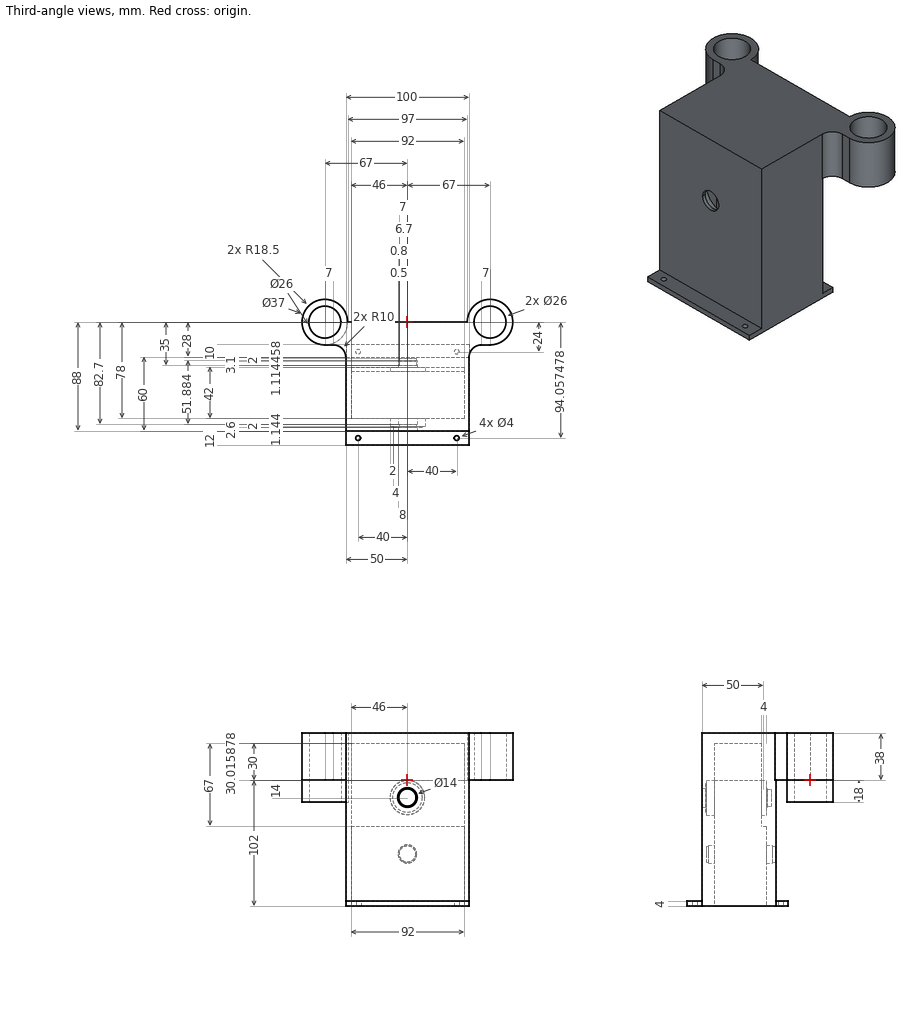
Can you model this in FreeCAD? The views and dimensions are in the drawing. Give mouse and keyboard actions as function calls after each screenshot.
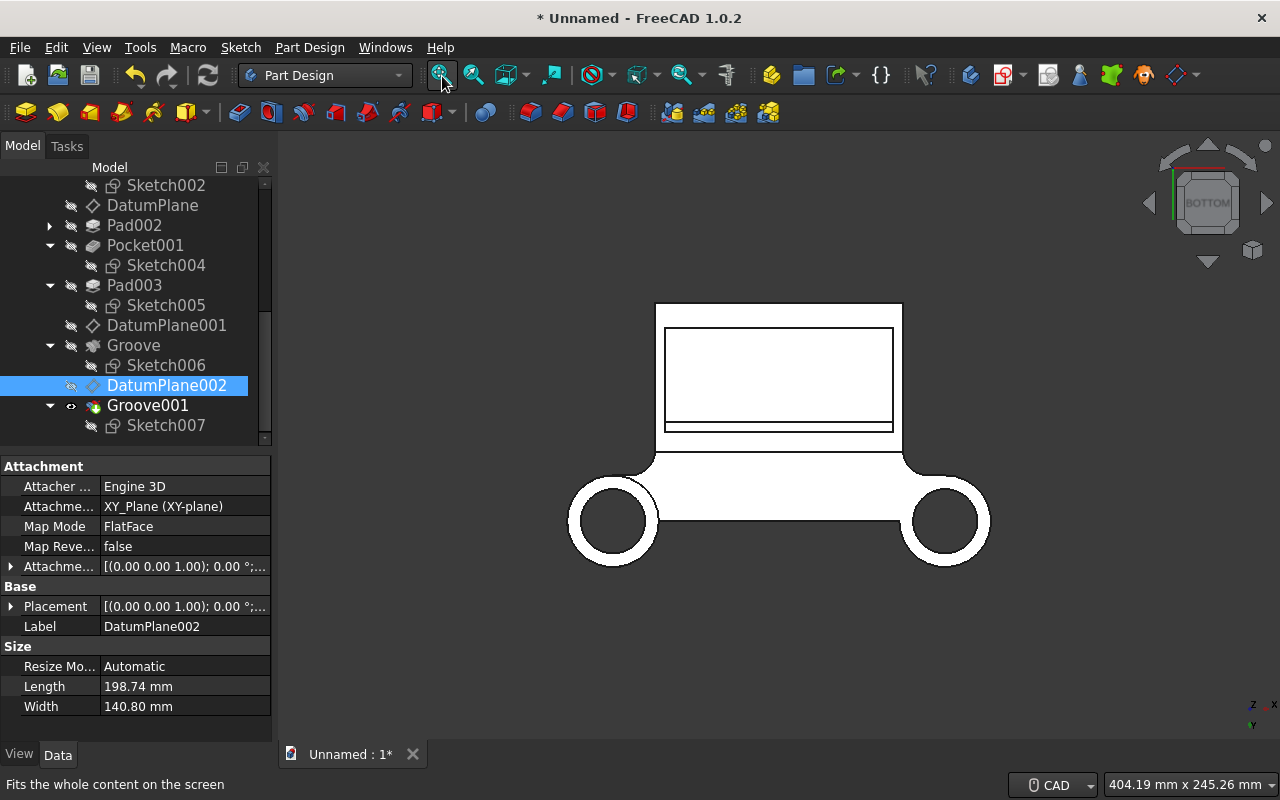
click(885, 313)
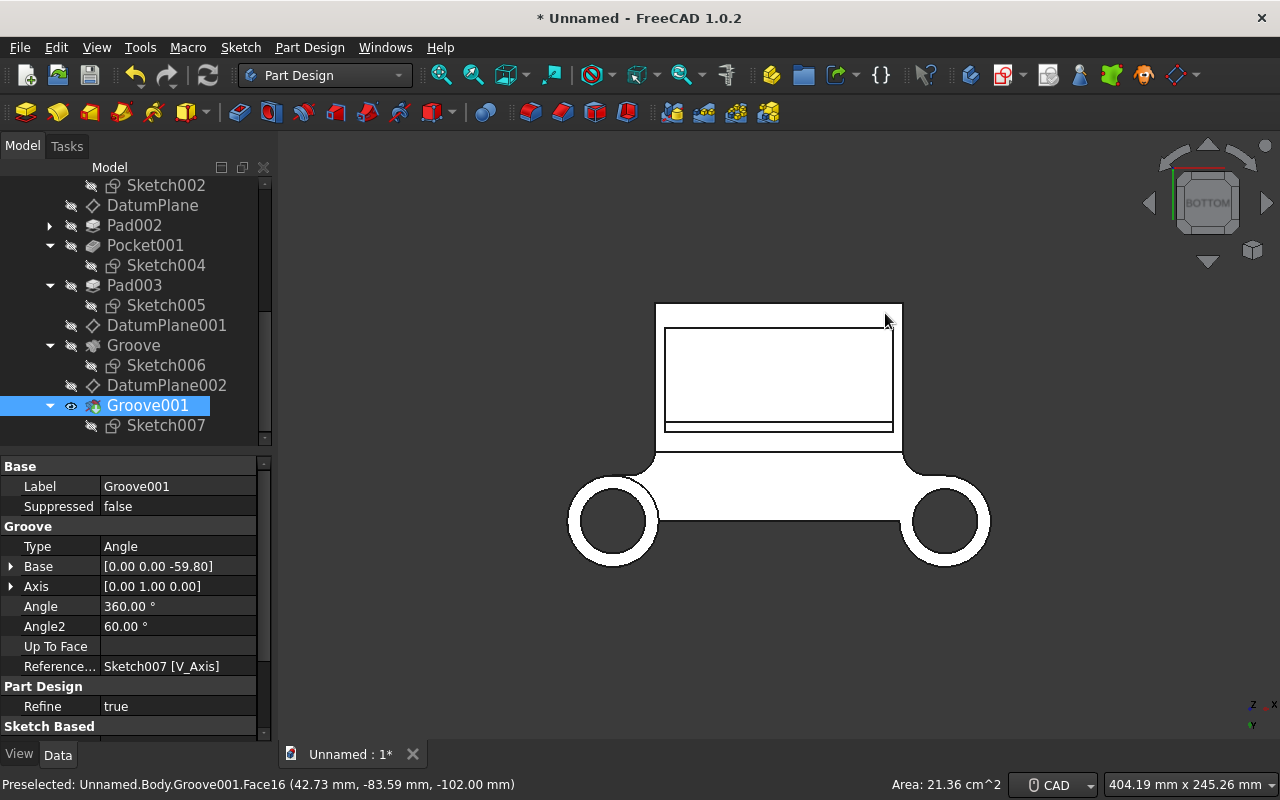
click(1004, 76)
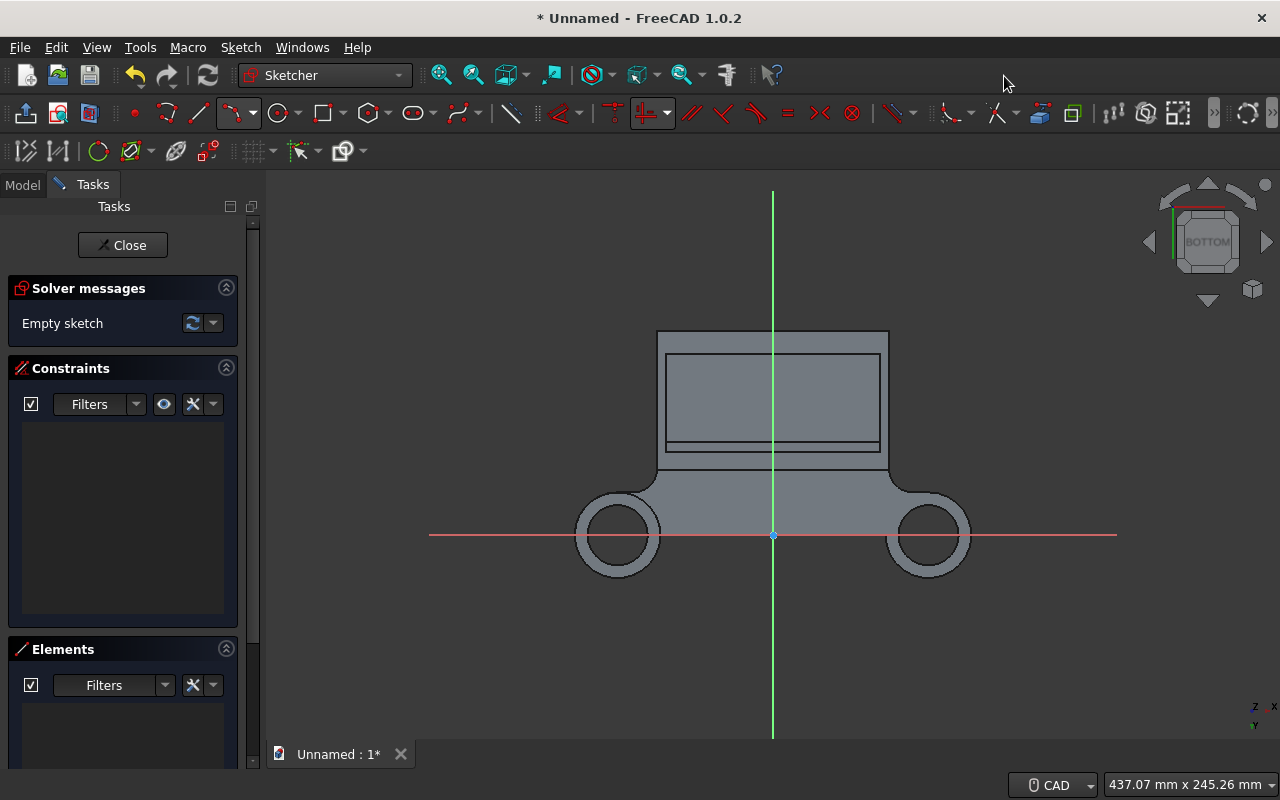
scroll(912, 347, up, 2)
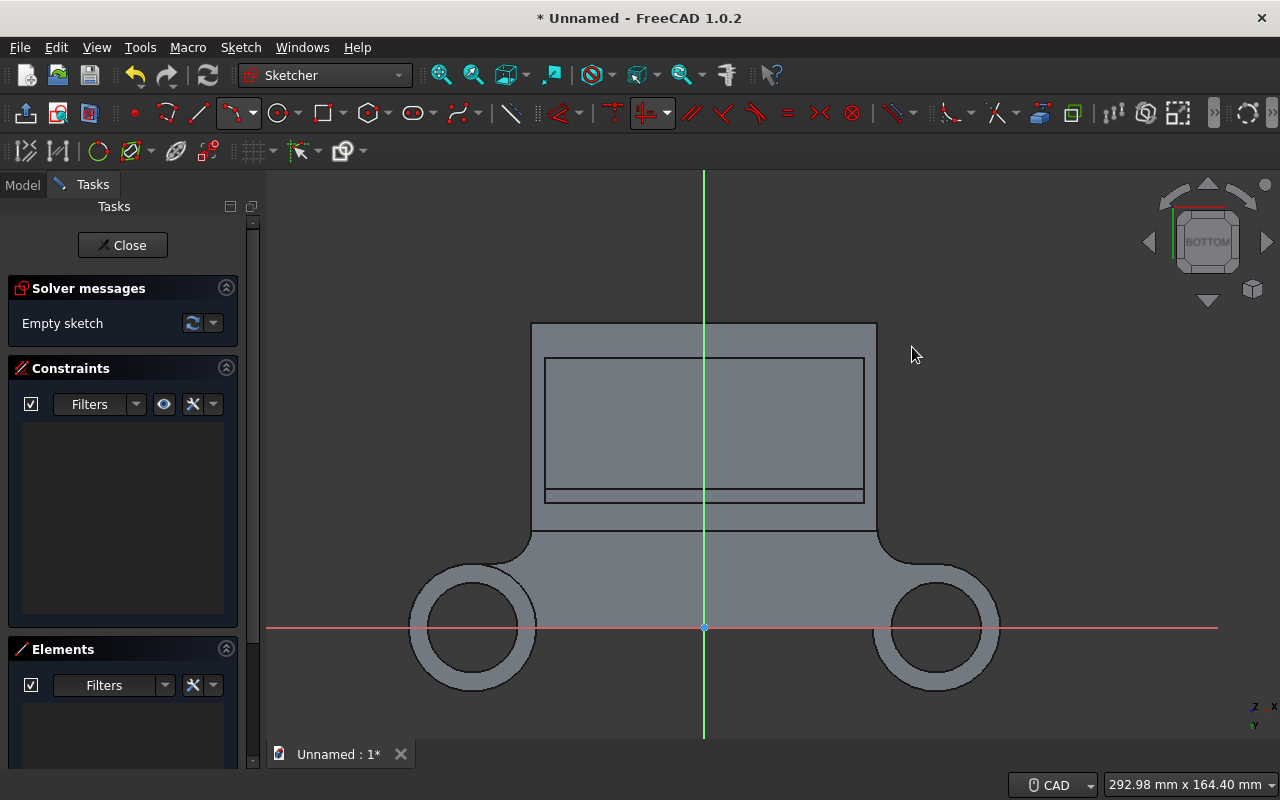
key(g)
key(r)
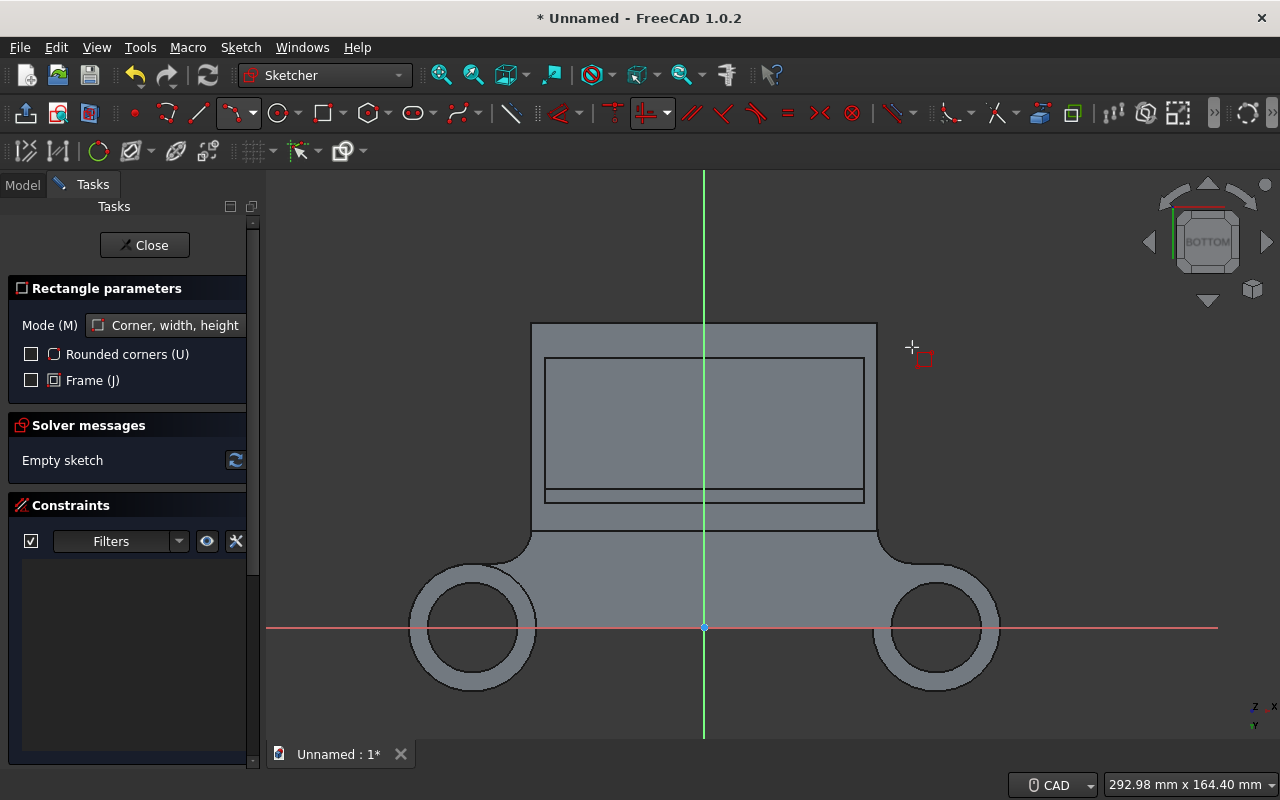
click(531, 531)
click(877, 565)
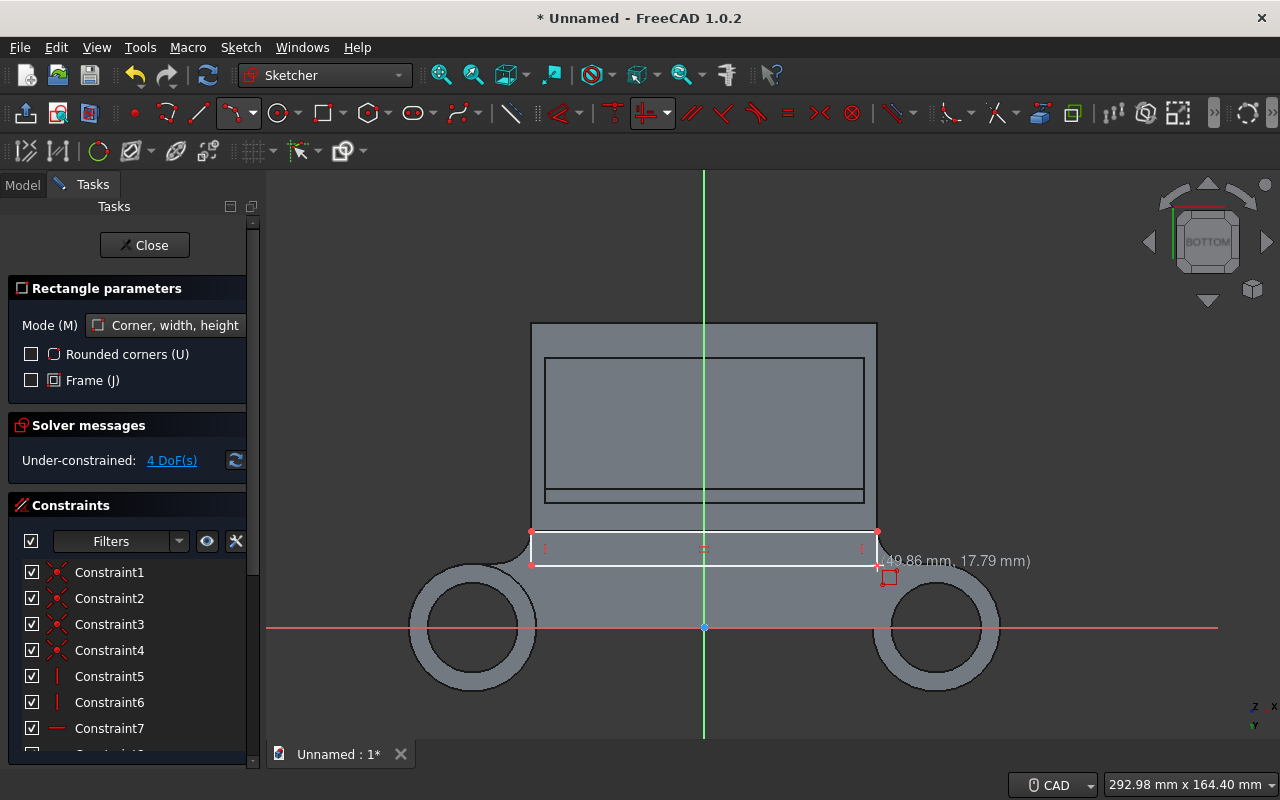
click(531, 281)
click(877, 323)
key(Escape)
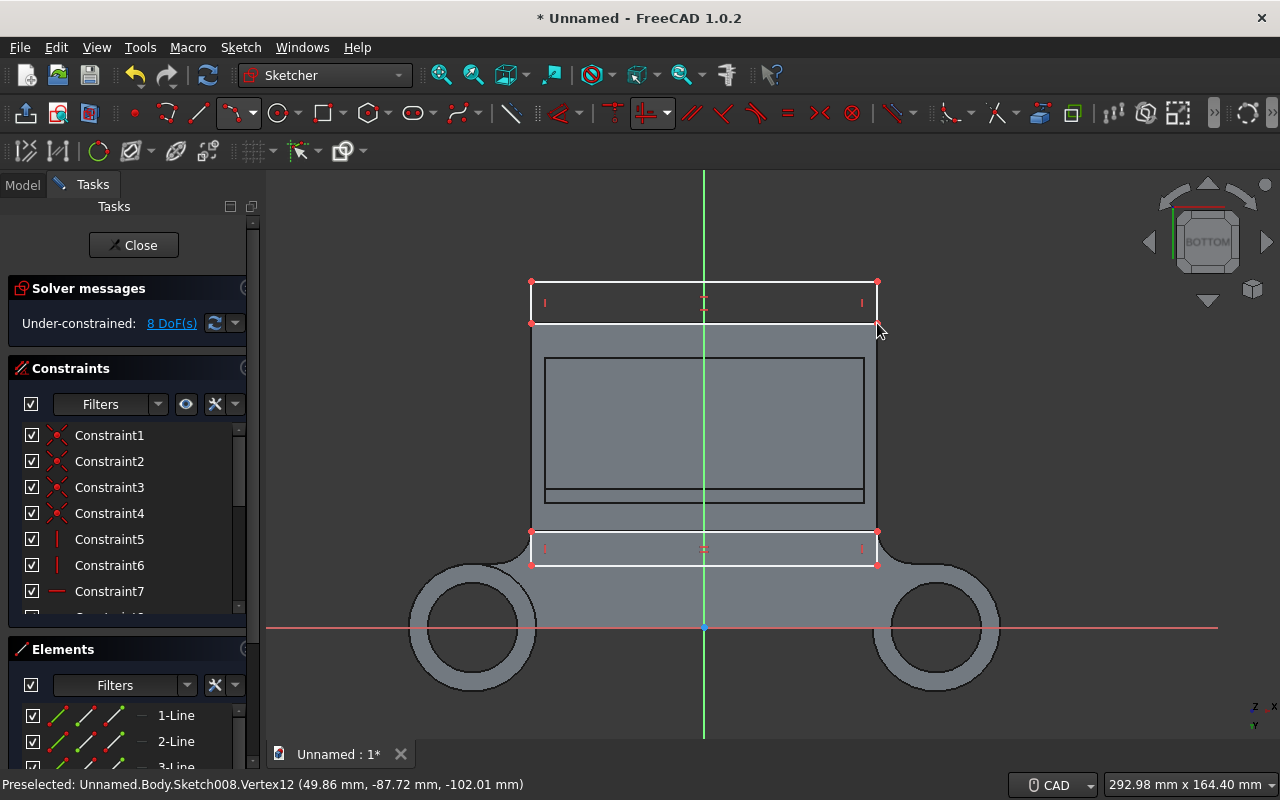
key(d)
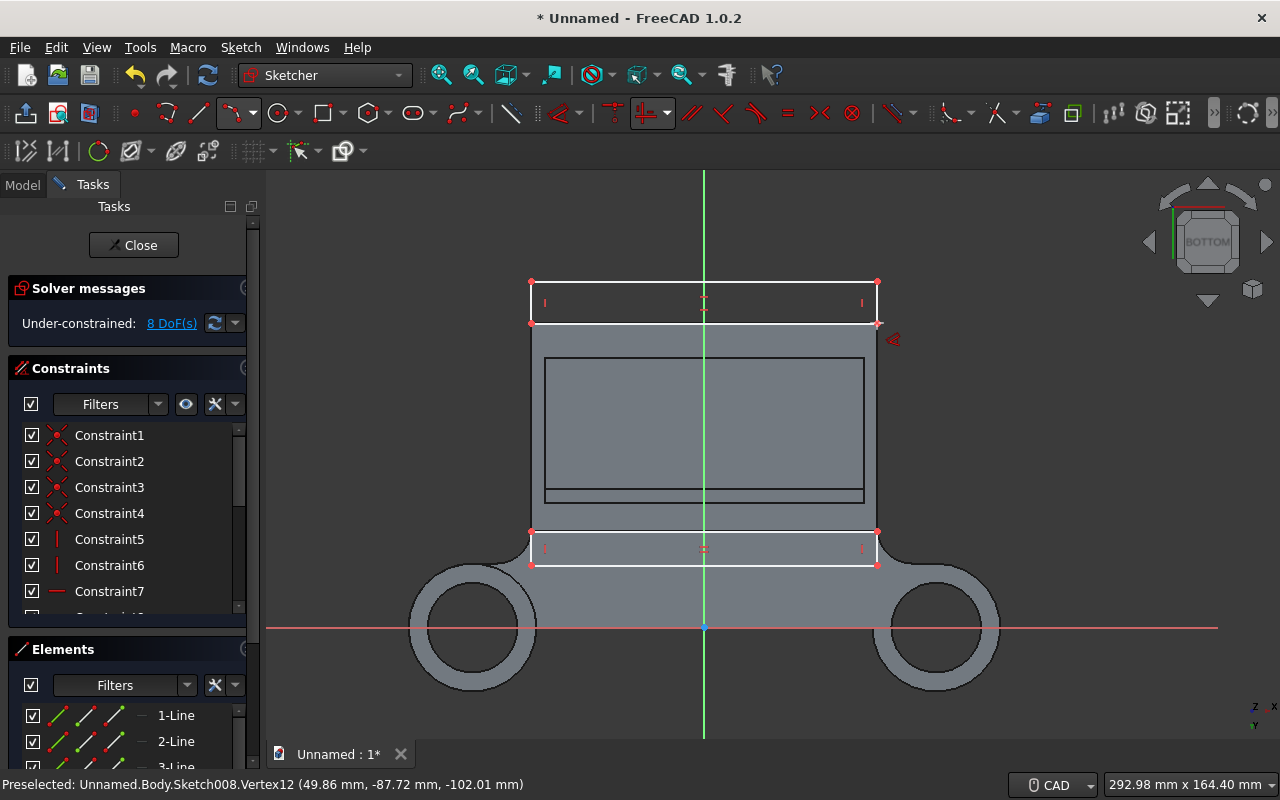
scroll(531, 542, up, 2)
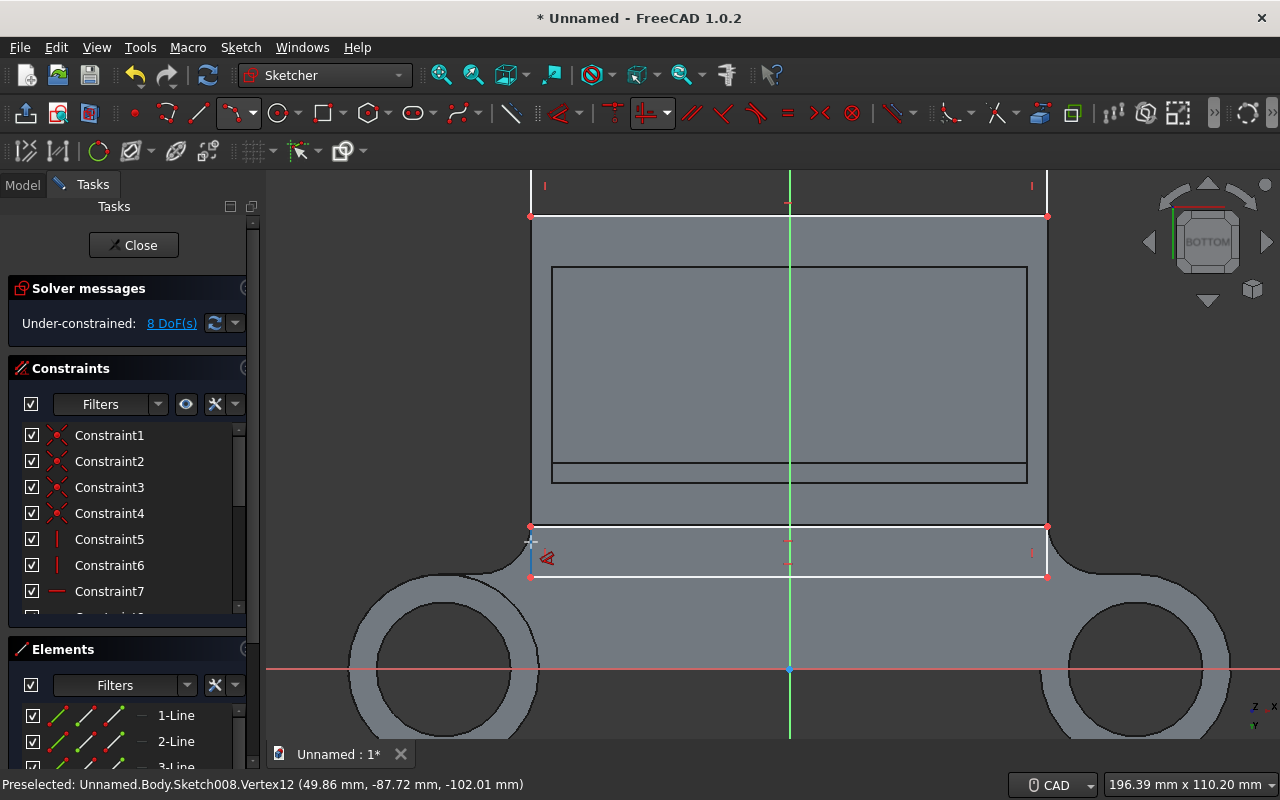
click(531, 542)
click(497, 552)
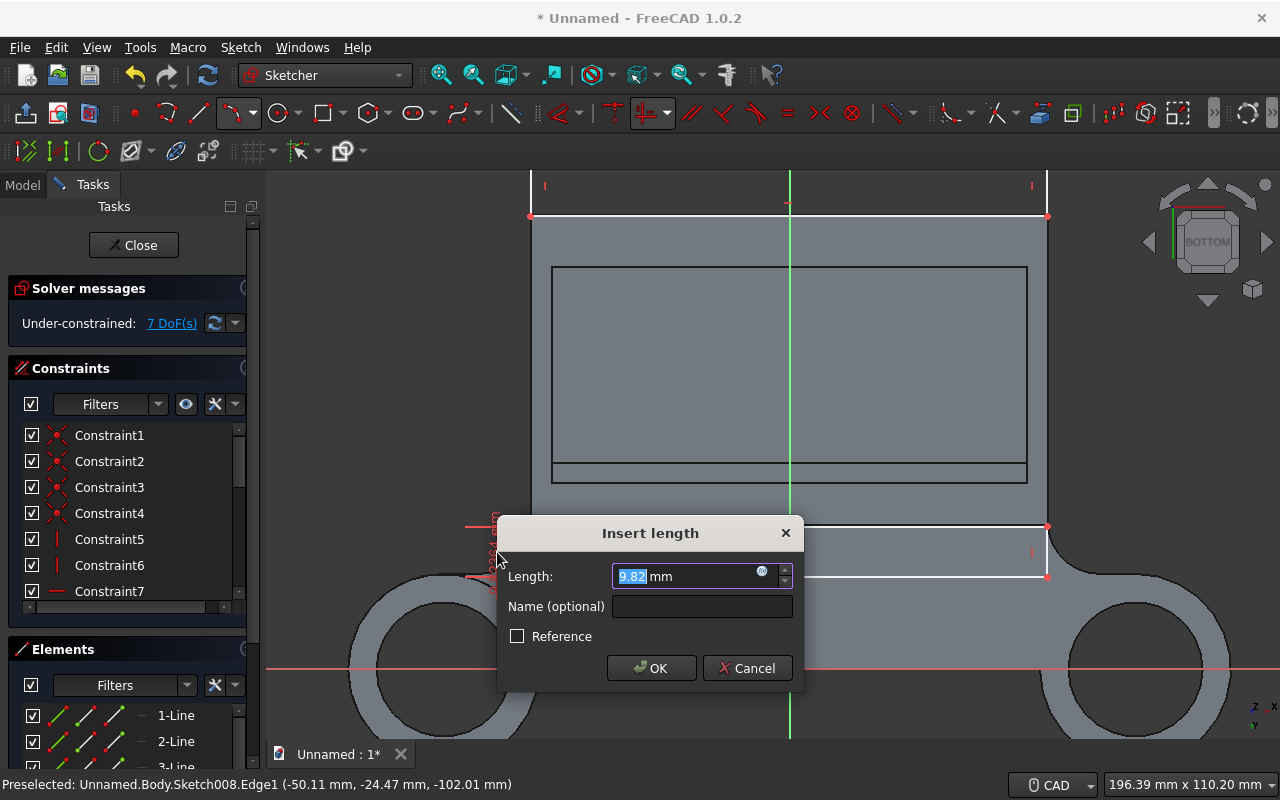
text(10)
key(Return)